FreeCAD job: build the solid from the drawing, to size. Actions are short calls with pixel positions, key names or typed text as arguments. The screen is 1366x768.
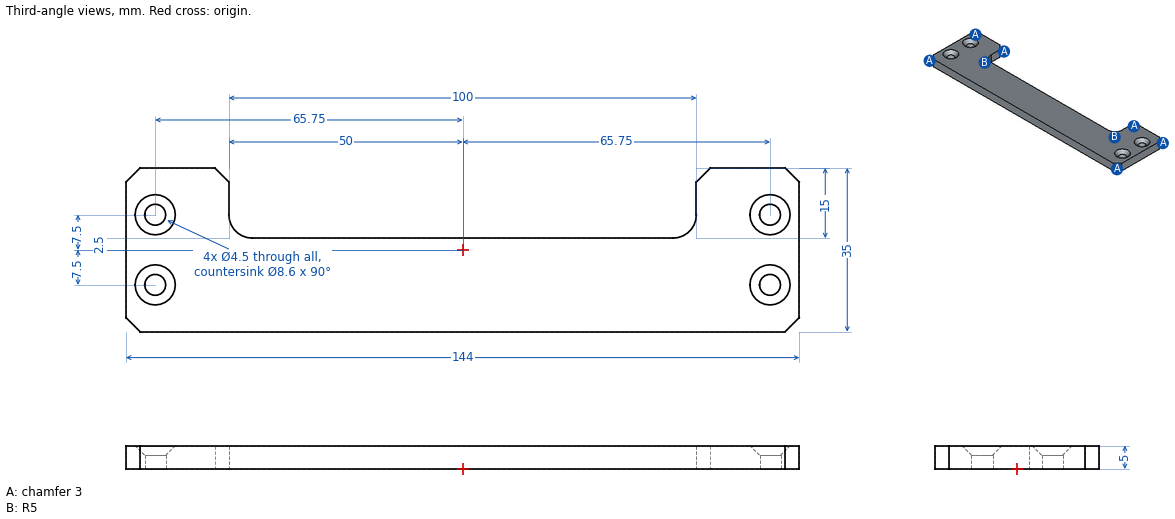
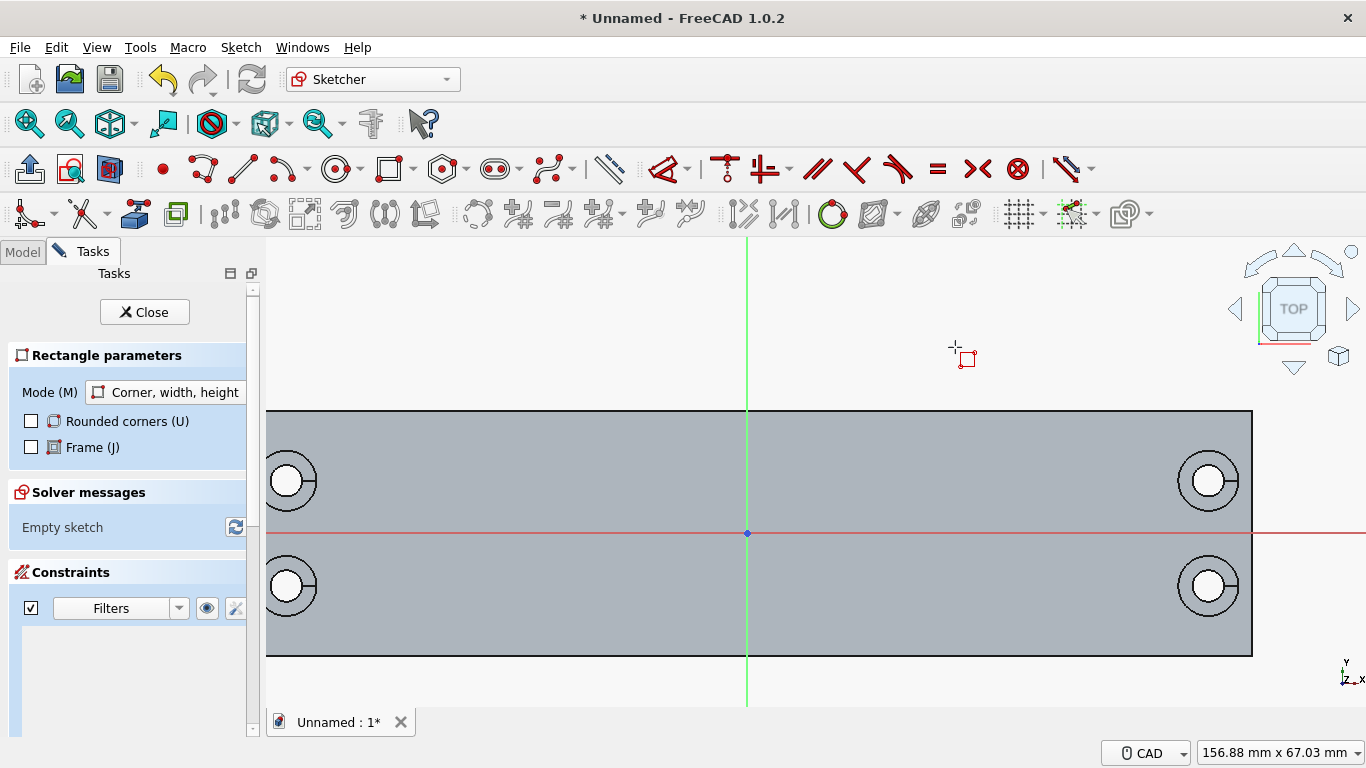
click(397, 411)
move(1098, 516)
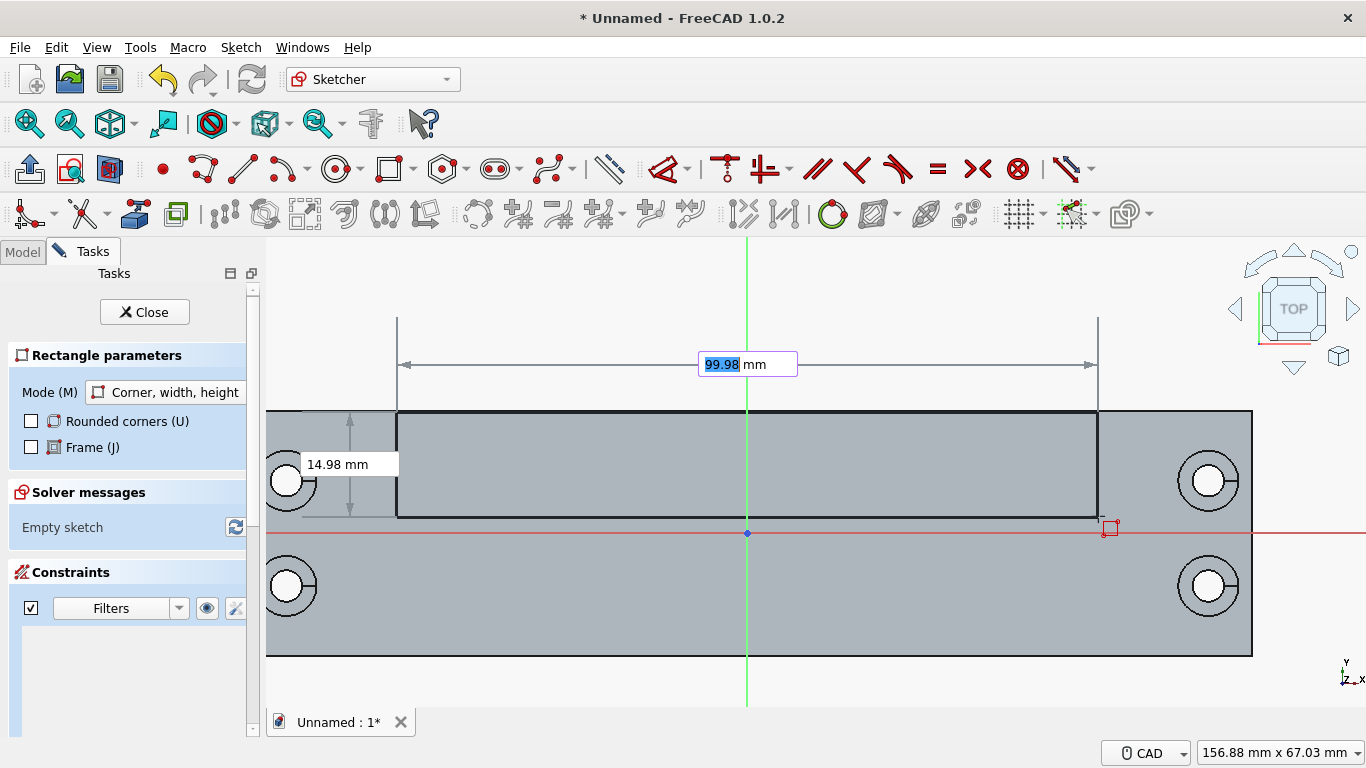
text(100)
key(Tab)
text(15)
key(Return)
key(Escape)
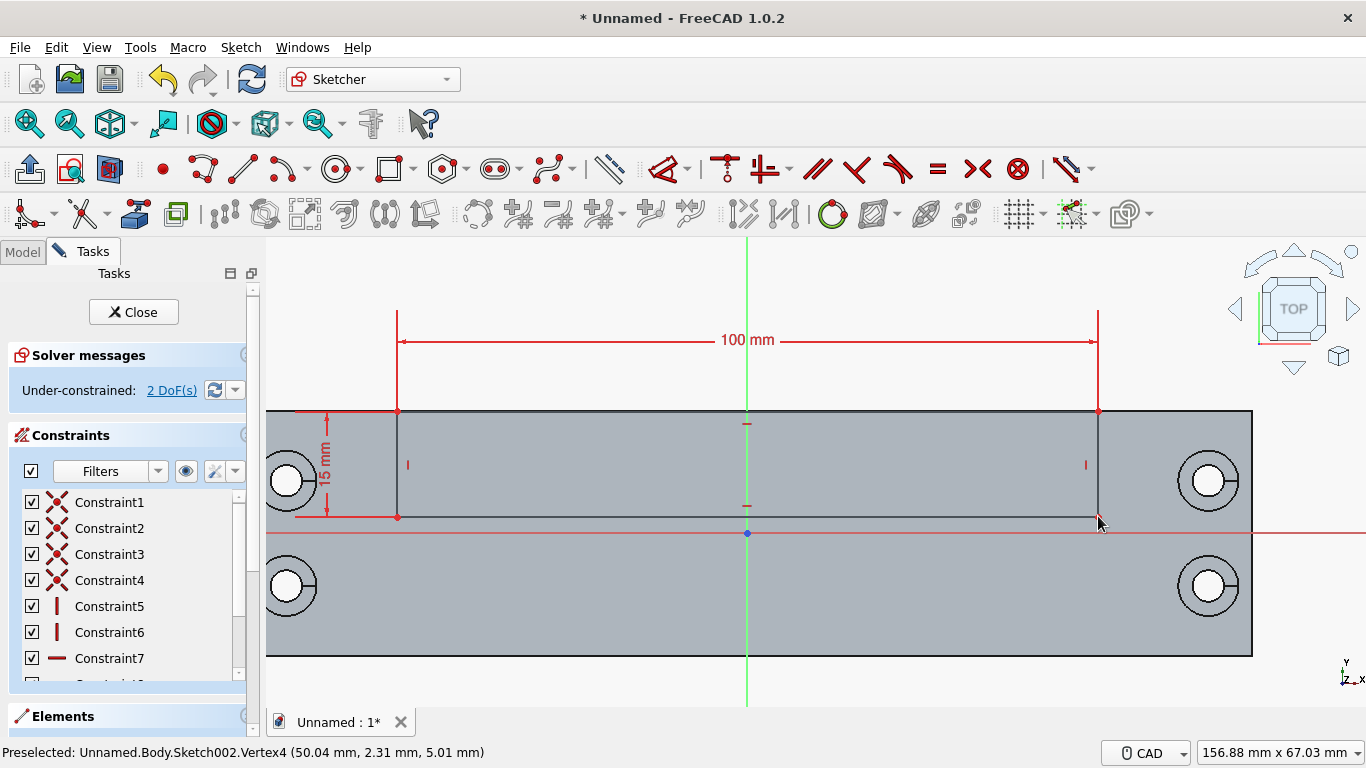
key(d)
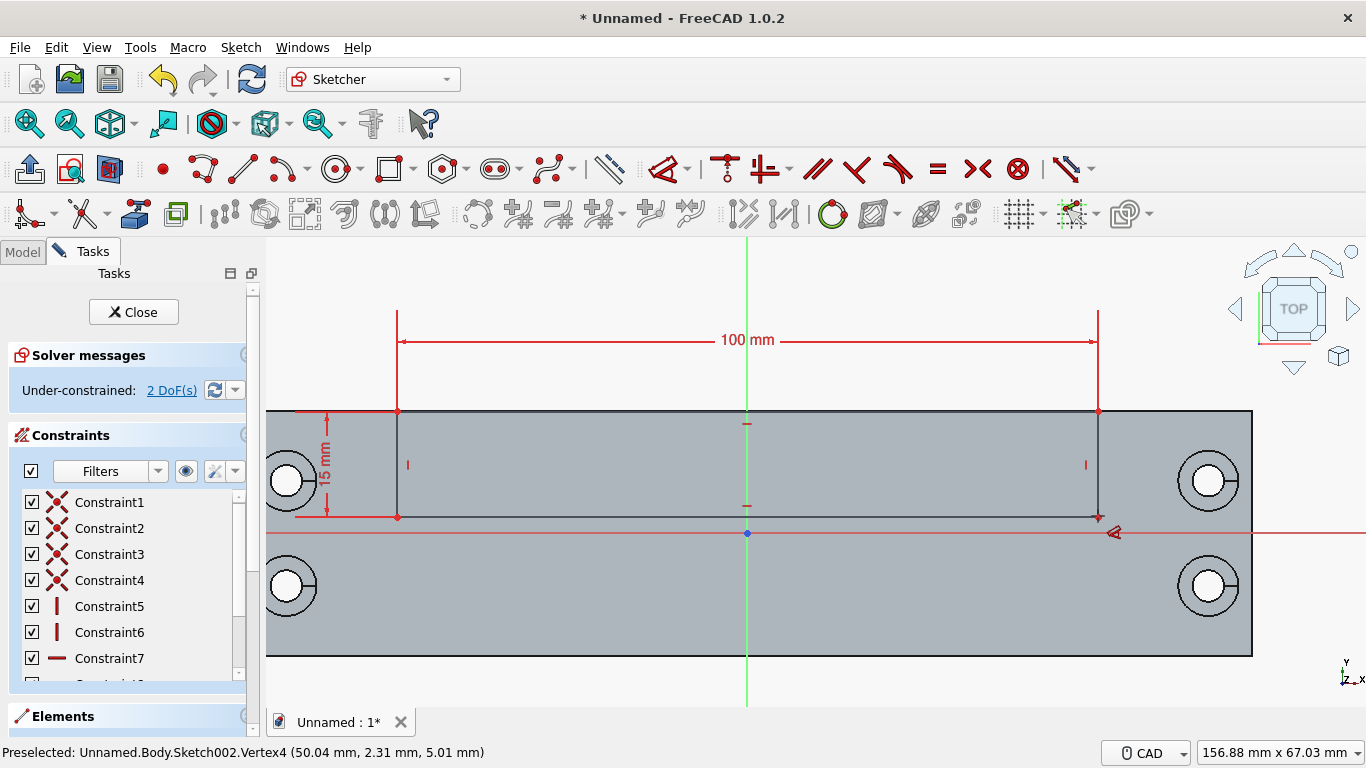
click(397, 412)
click(572, 567)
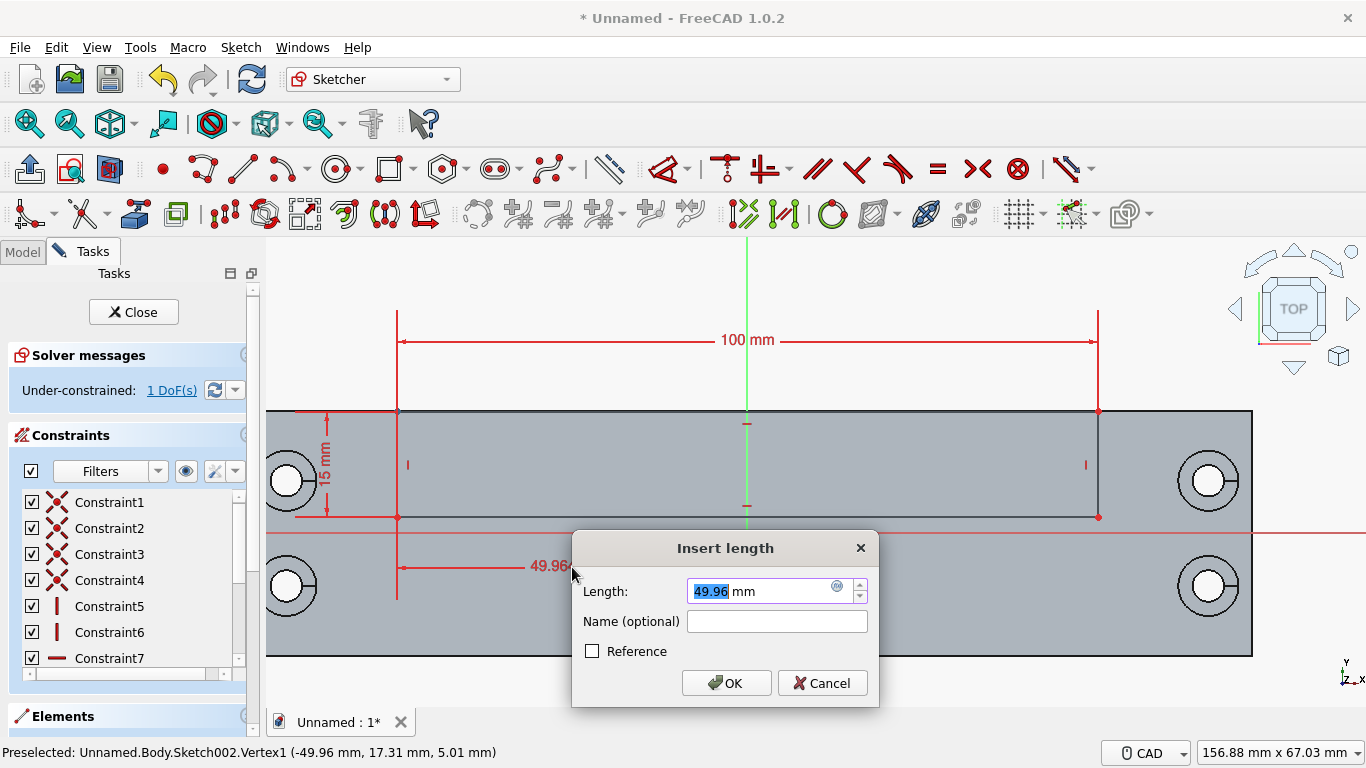
text(50)
key(Return)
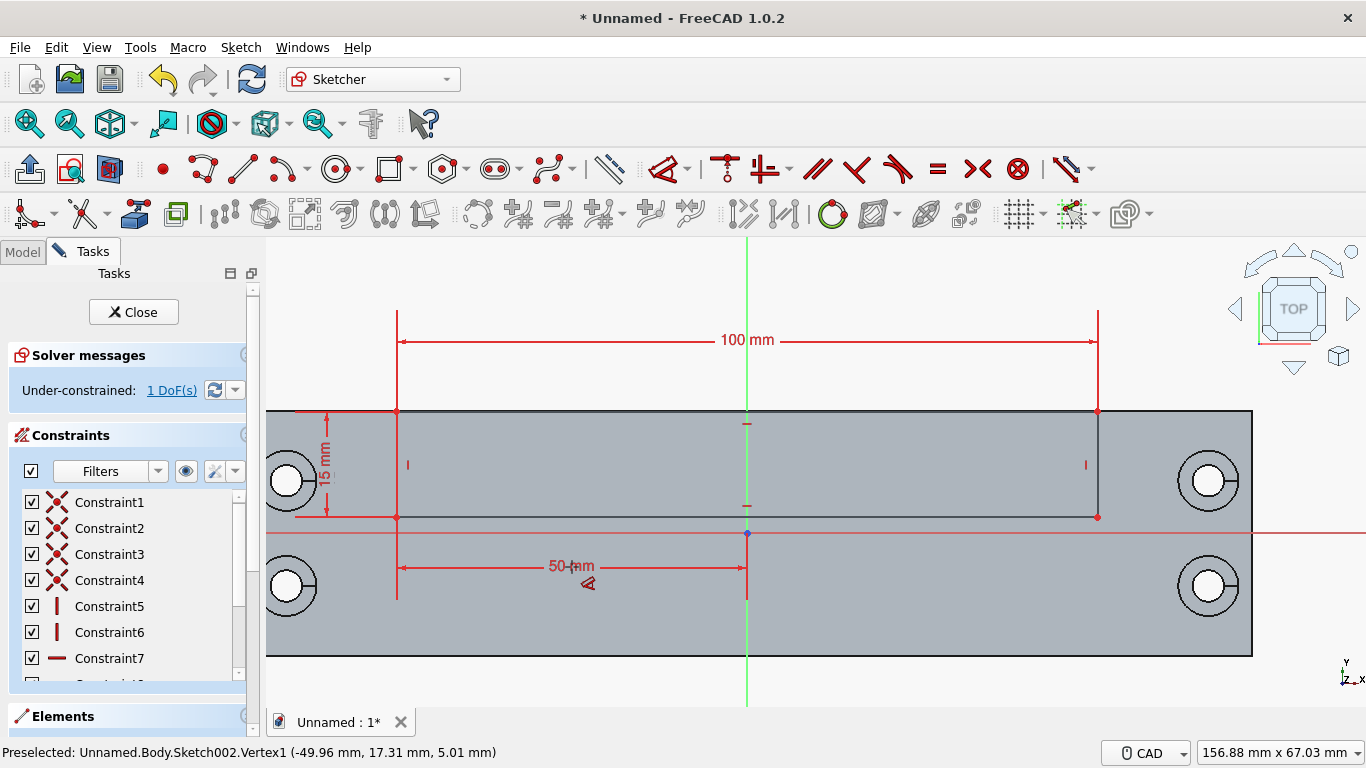
scroll(397, 517, up, 5)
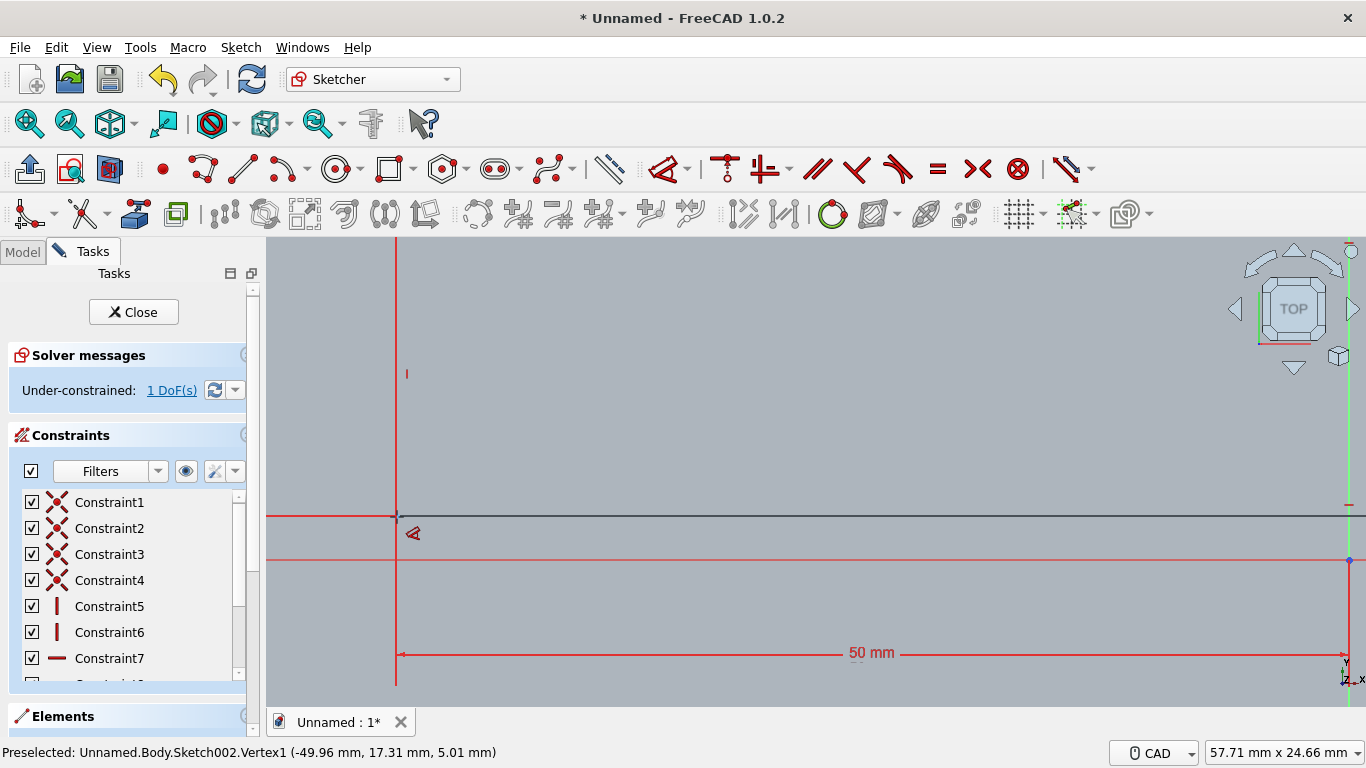
click(396, 516)
click(362, 538)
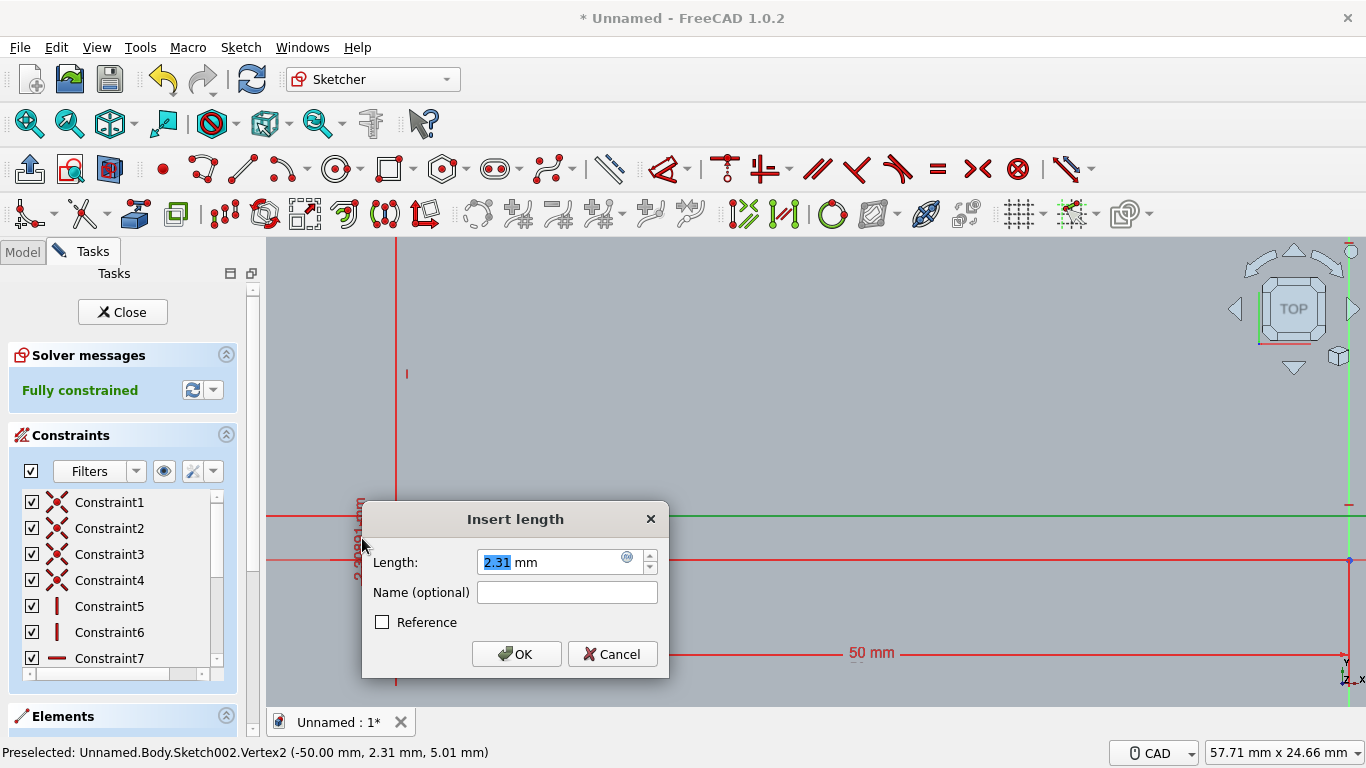
text(2.5)
key(Return)
key(Escape)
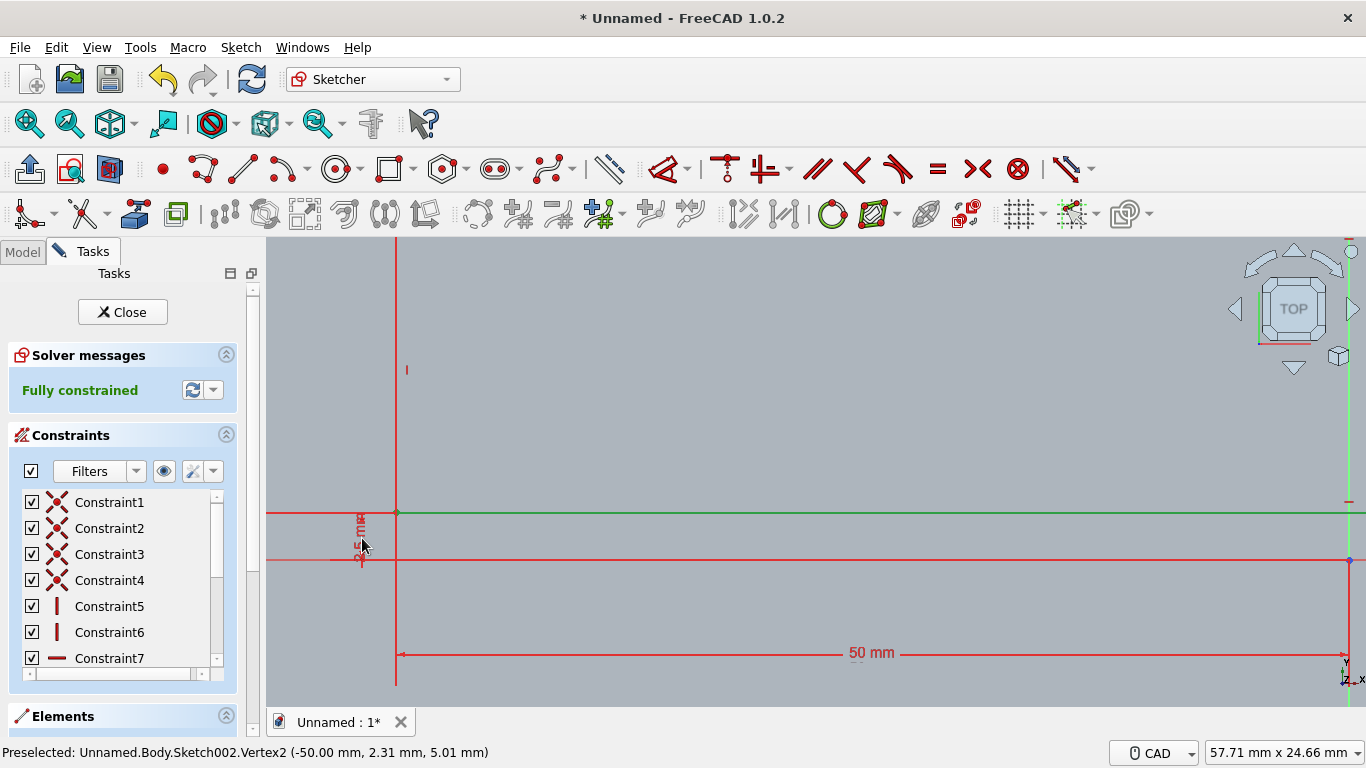
click(123, 312)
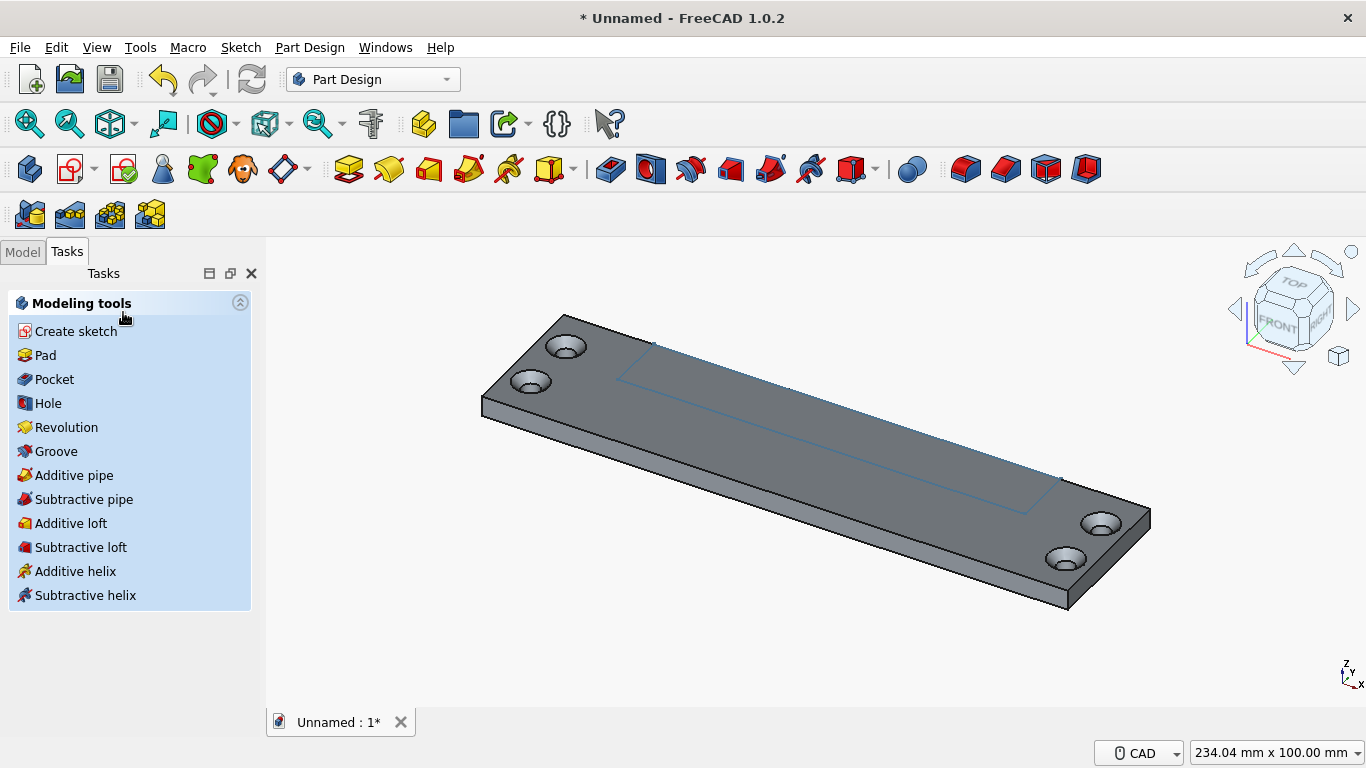
click(612, 170)